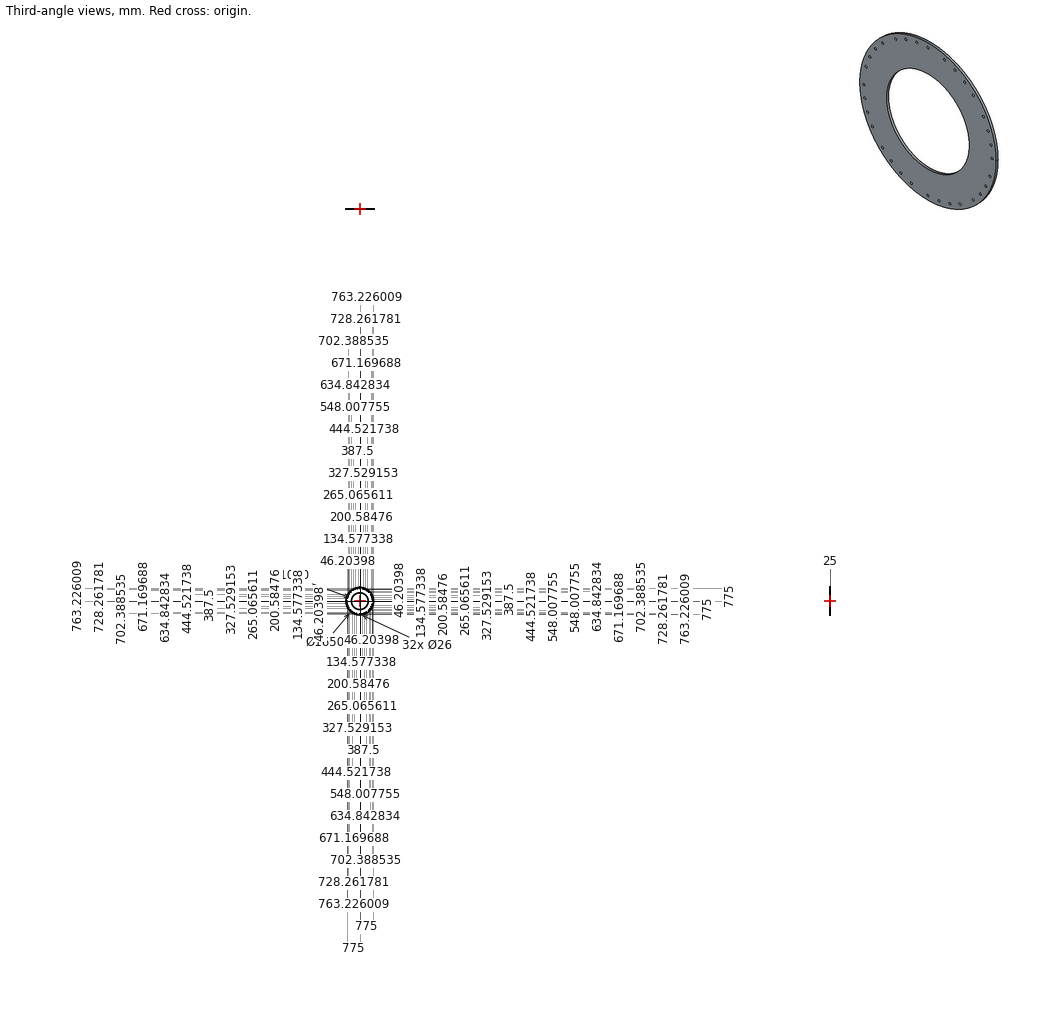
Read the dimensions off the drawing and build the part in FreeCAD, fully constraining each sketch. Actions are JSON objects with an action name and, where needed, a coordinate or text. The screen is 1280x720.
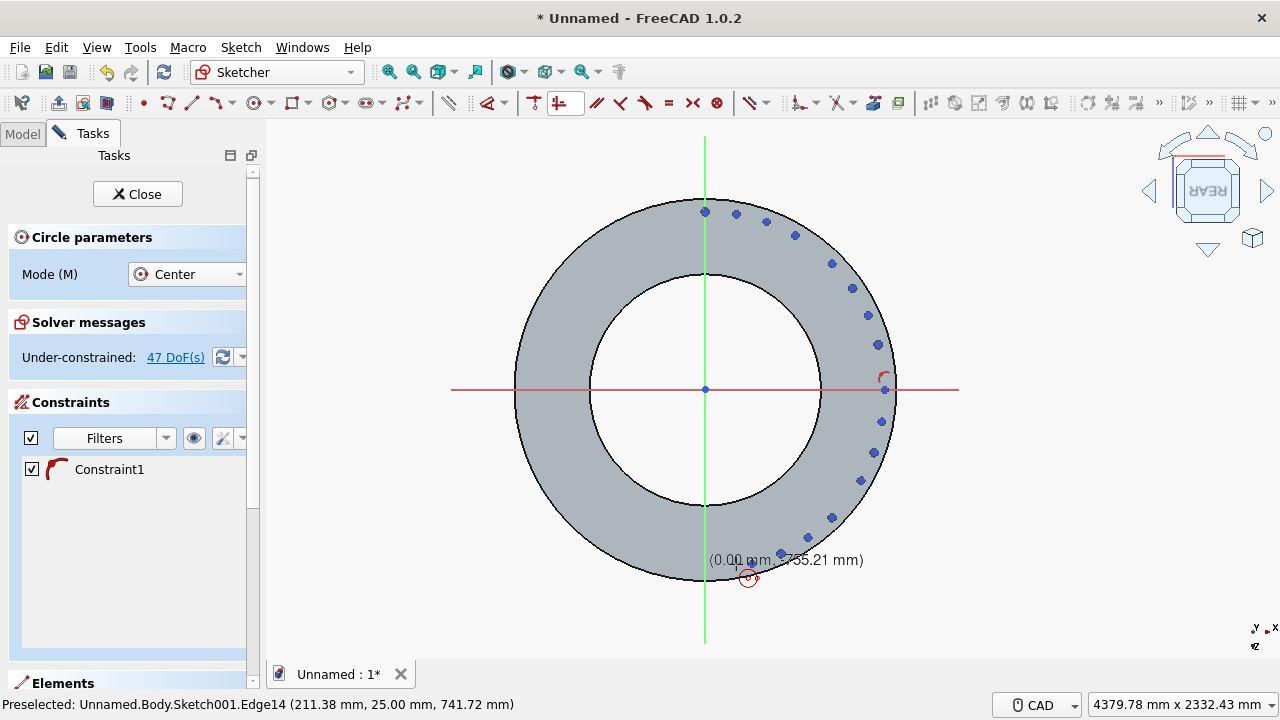
{"action": "left_click", "coordinate": [705, 569]}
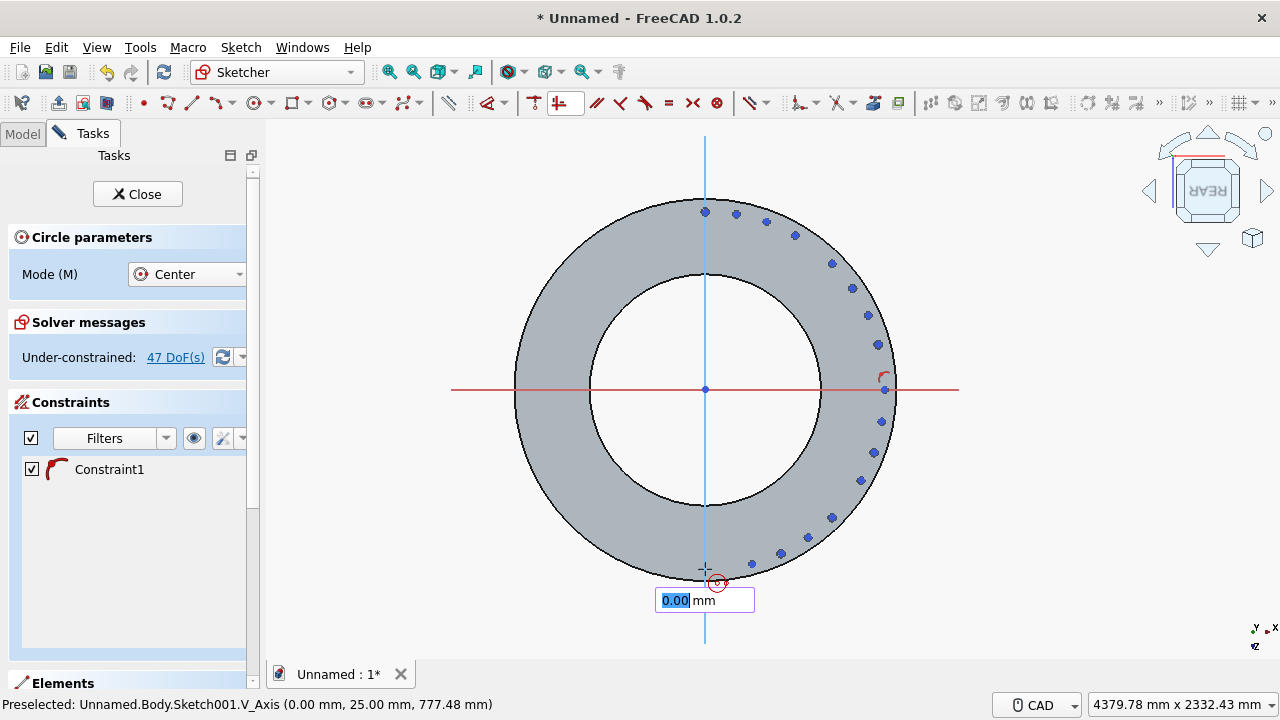
{"action": "scroll", "coordinate": [708, 568], "scroll_direction": "up", "scroll_amount": 9}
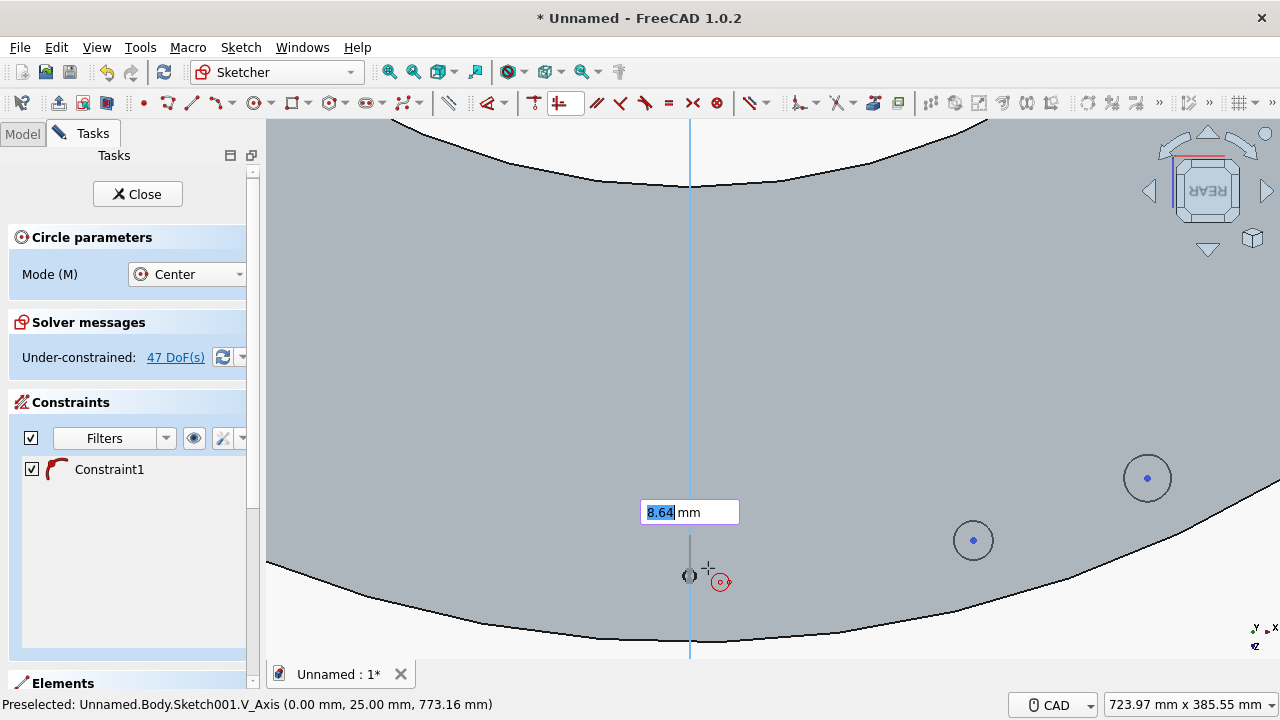
{"action": "left_click", "coordinate": [707, 566]}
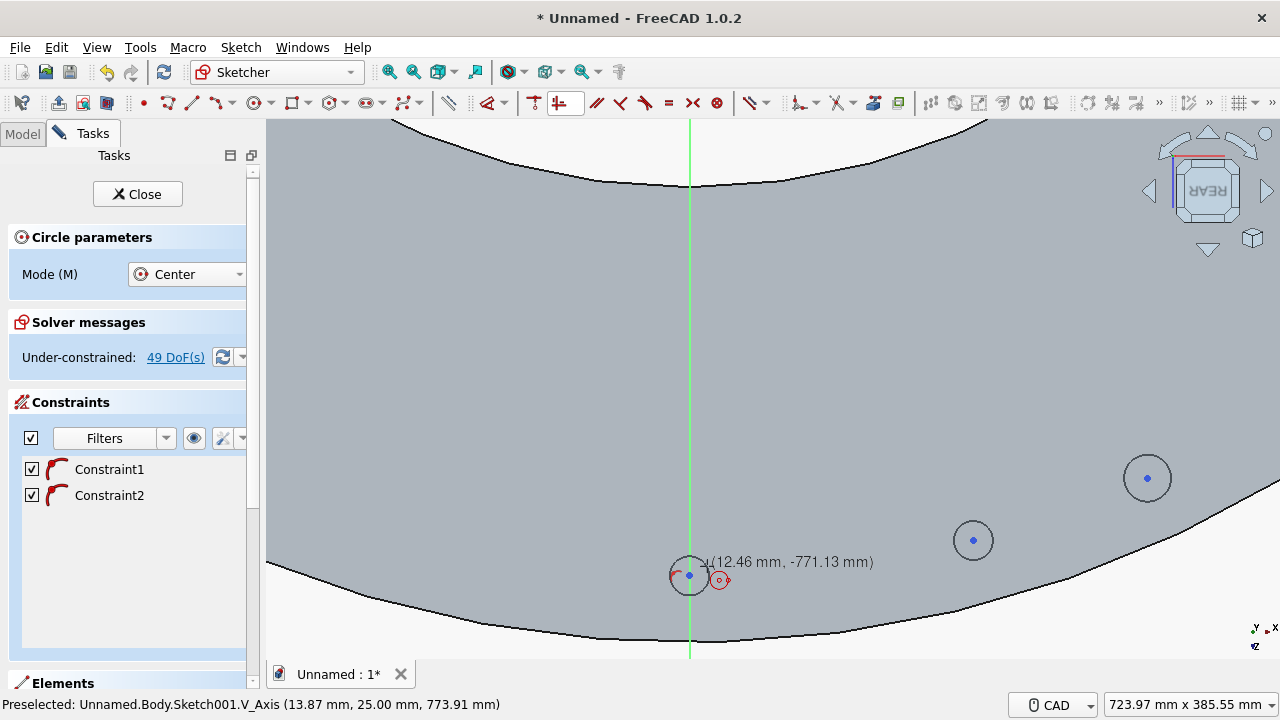
{"action": "scroll", "coordinate": [501, 556], "scroll_direction": "up", "scroll_amount": 2}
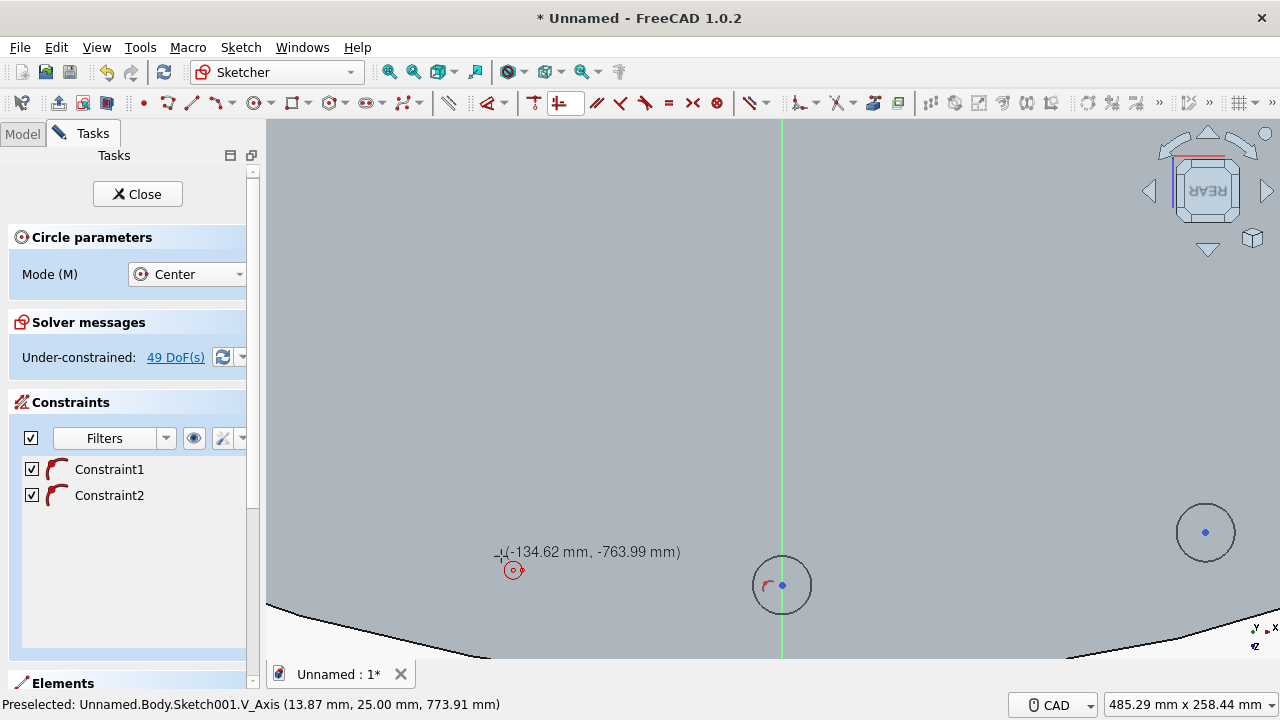
{"action": "scroll", "coordinate": [695, 567], "scroll_direction": "down", "scroll_amount": 11}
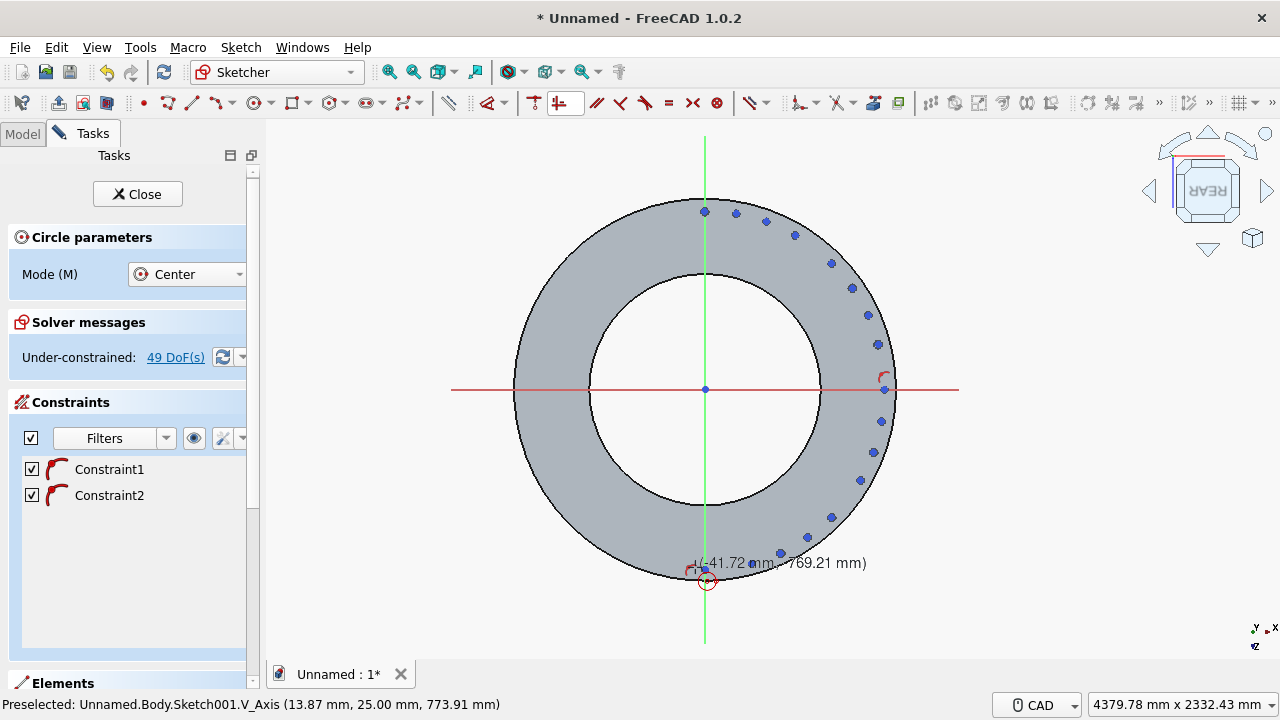
{"action": "left_click", "coordinate": [674, 566]}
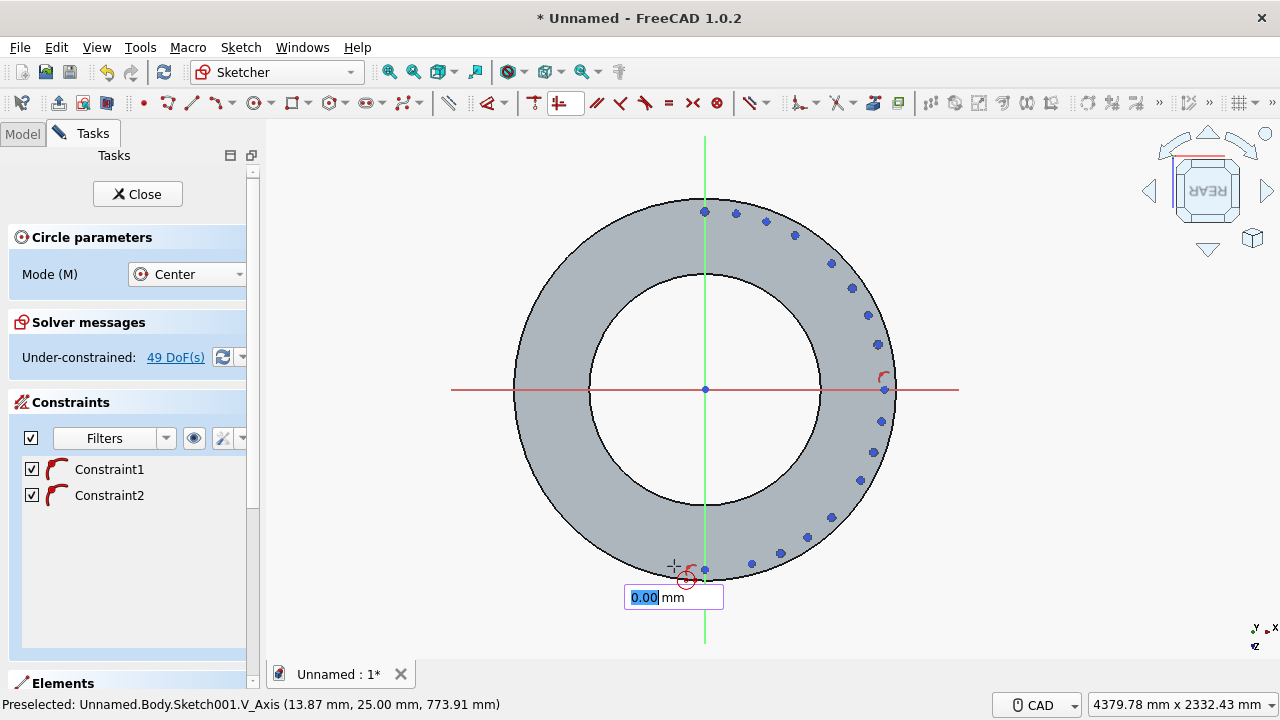
{"action": "scroll", "coordinate": [676, 564], "scroll_direction": "up", "scroll_amount": 9}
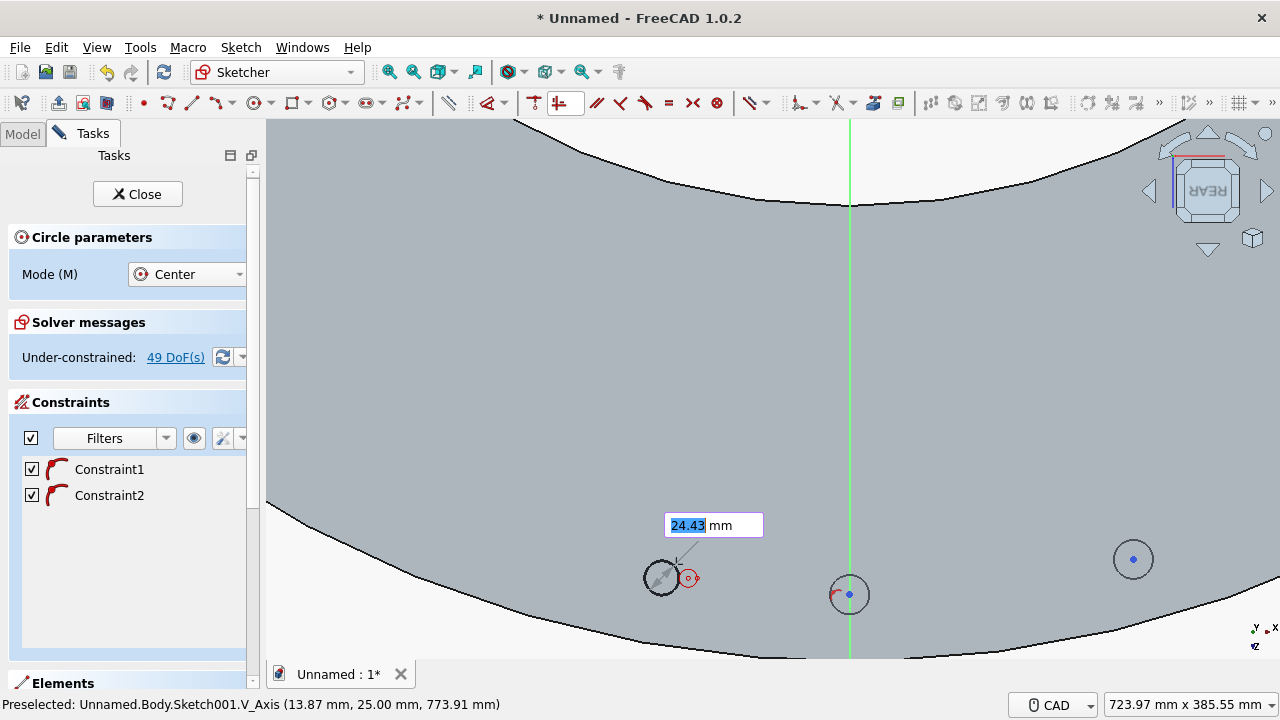
{"action": "left_click", "coordinate": [674, 562]}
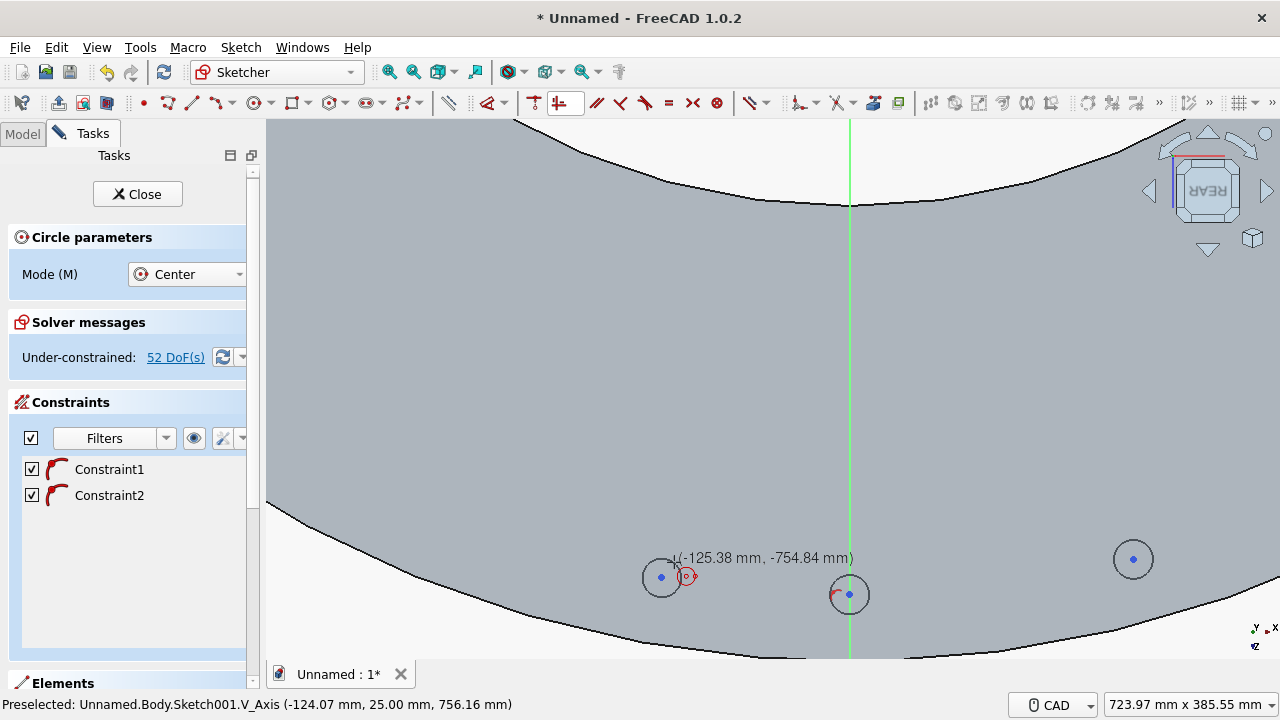
{"action": "scroll", "coordinate": [478, 526], "scroll_direction": "up", "scroll_amount": 2}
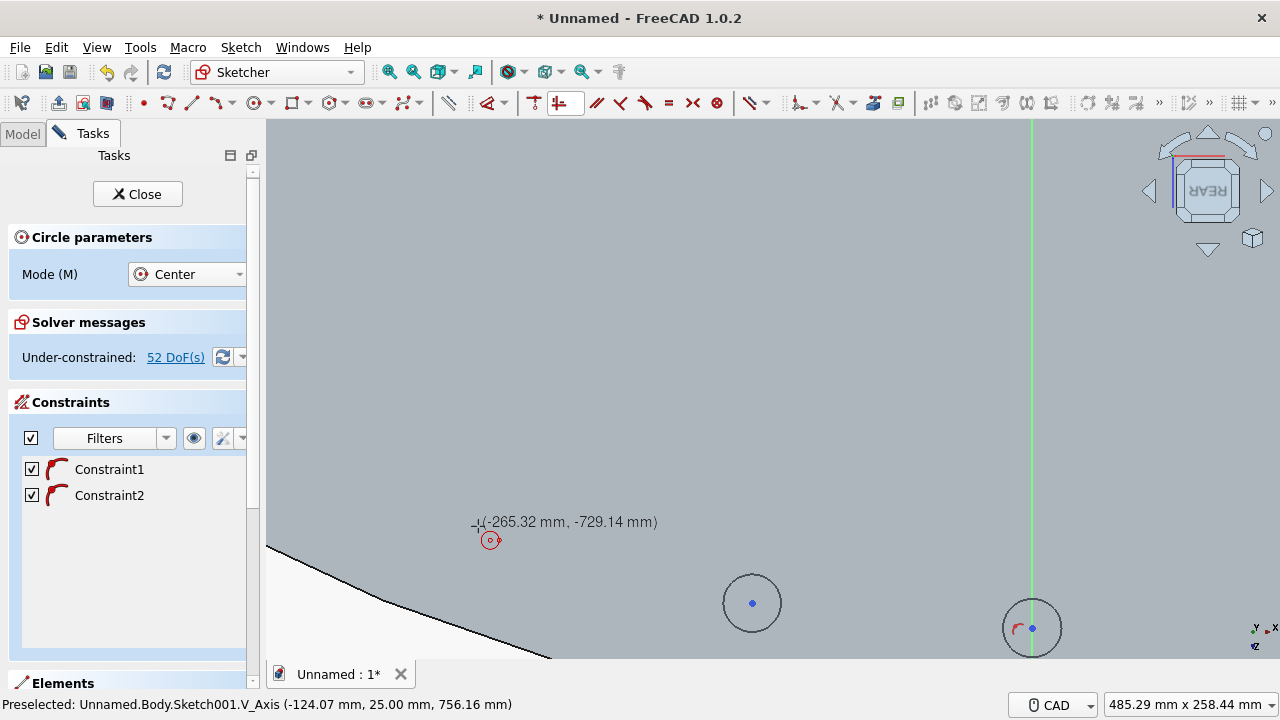
{"action": "scroll", "coordinate": [664, 562], "scroll_direction": "down", "scroll_amount": 11}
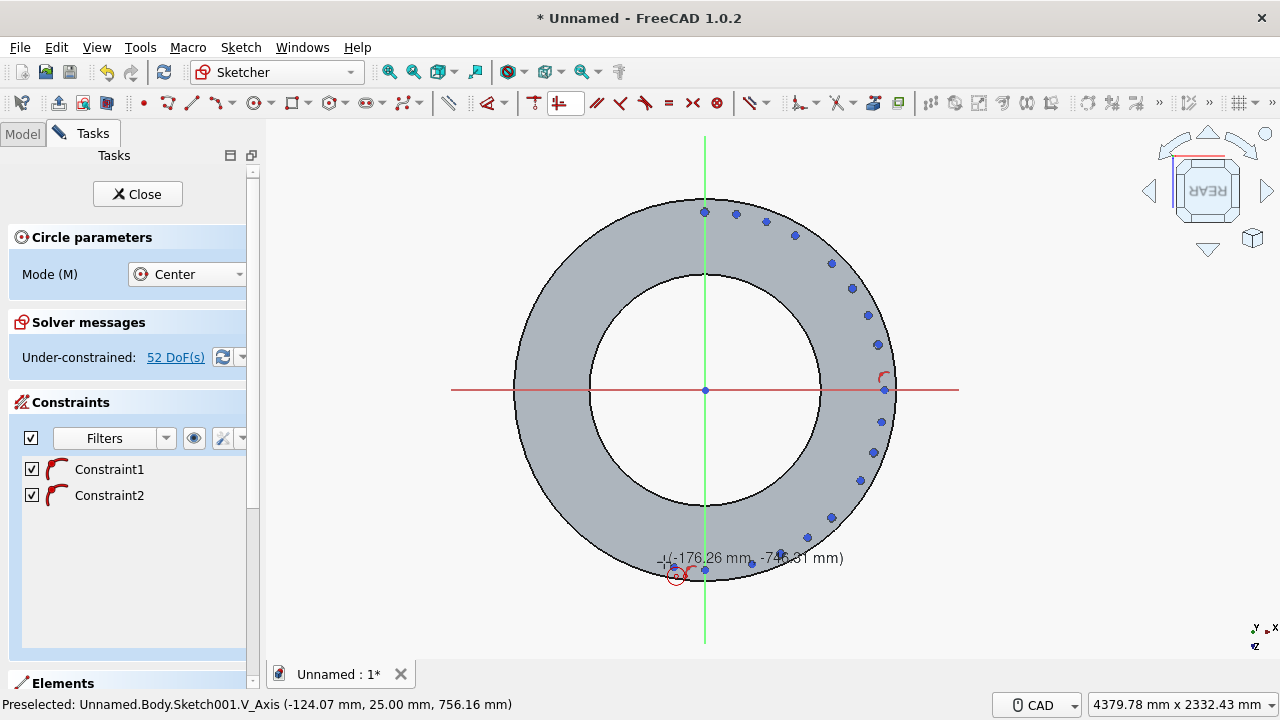
{"action": "left_click", "coordinate": [644, 559]}